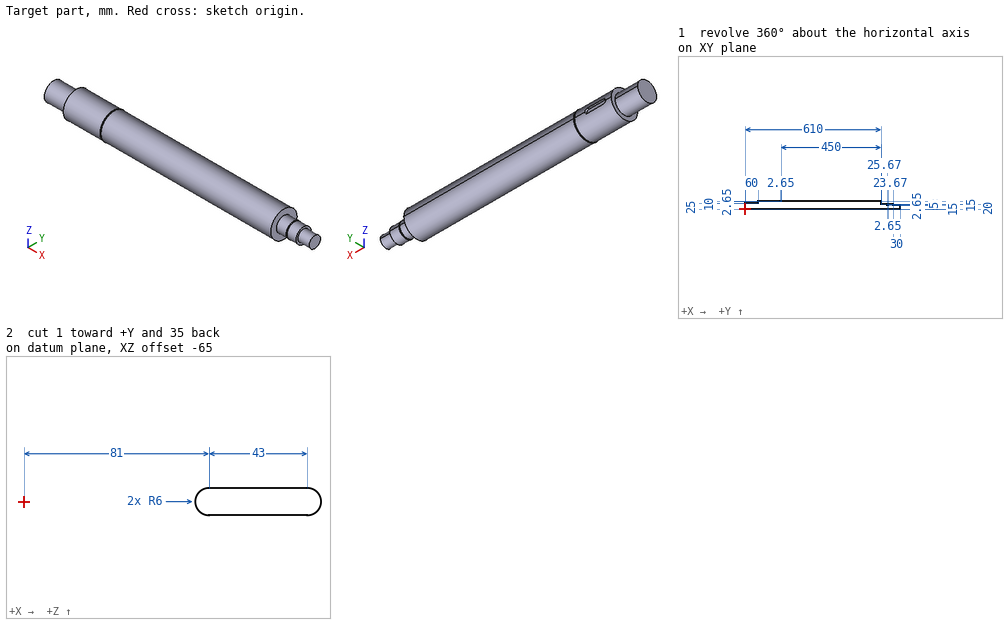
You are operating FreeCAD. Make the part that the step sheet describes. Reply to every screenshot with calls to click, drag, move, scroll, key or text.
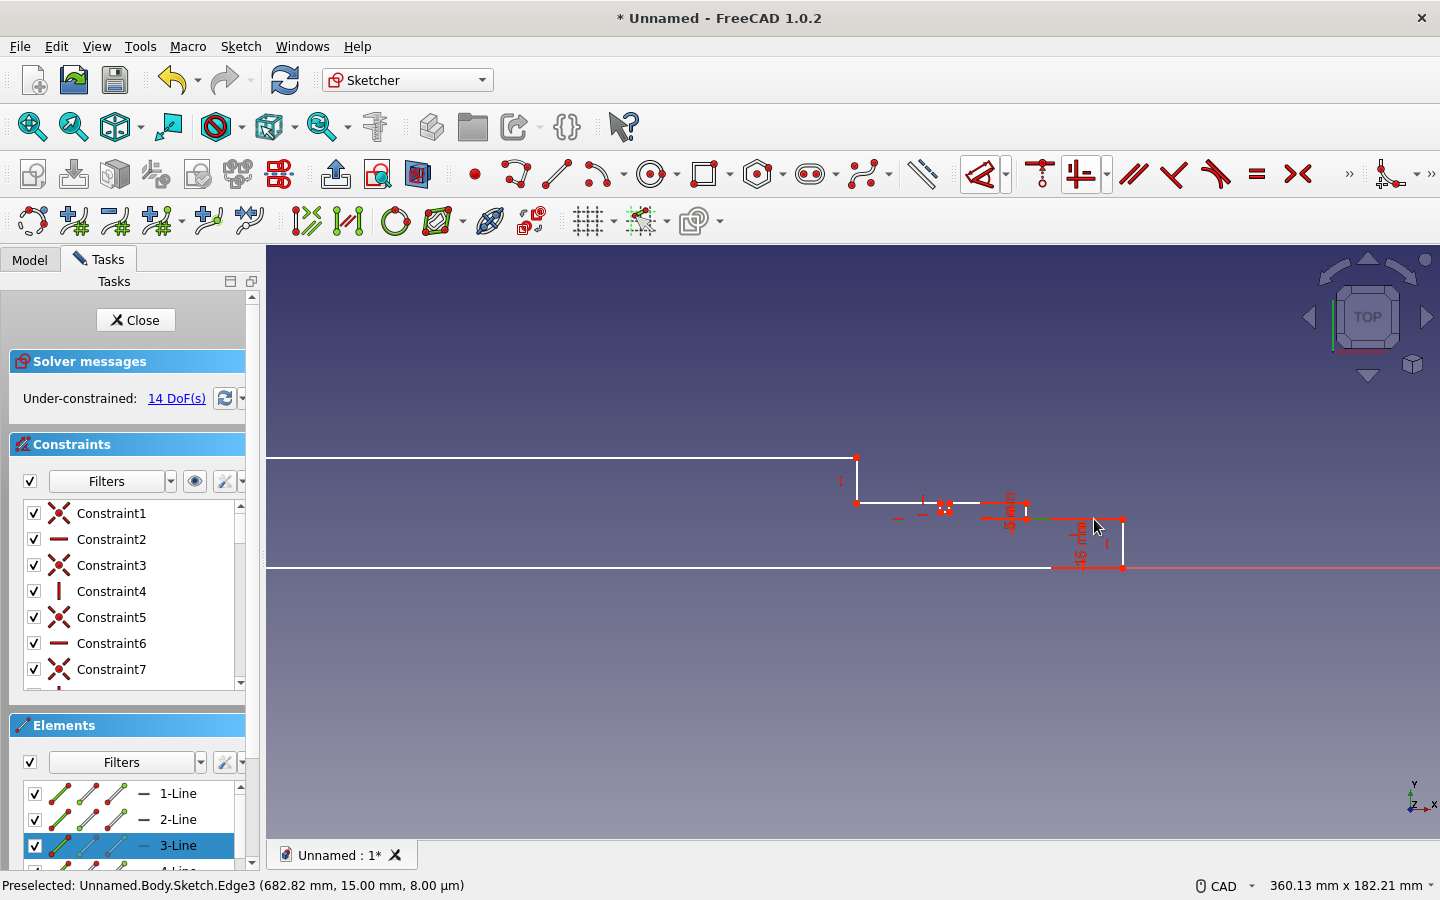
key(l)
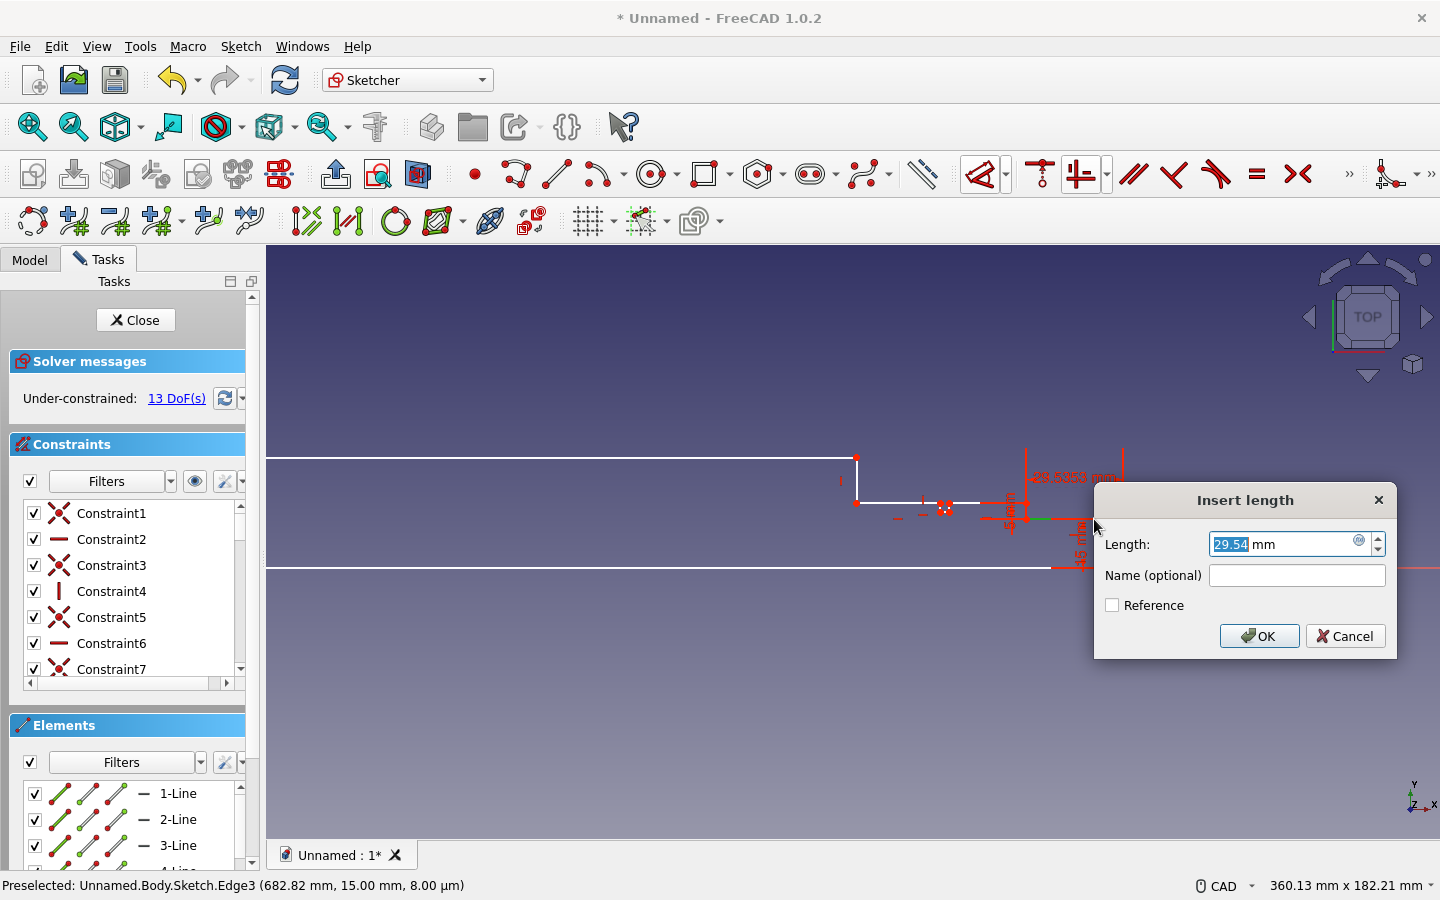
text(30)
key(Return)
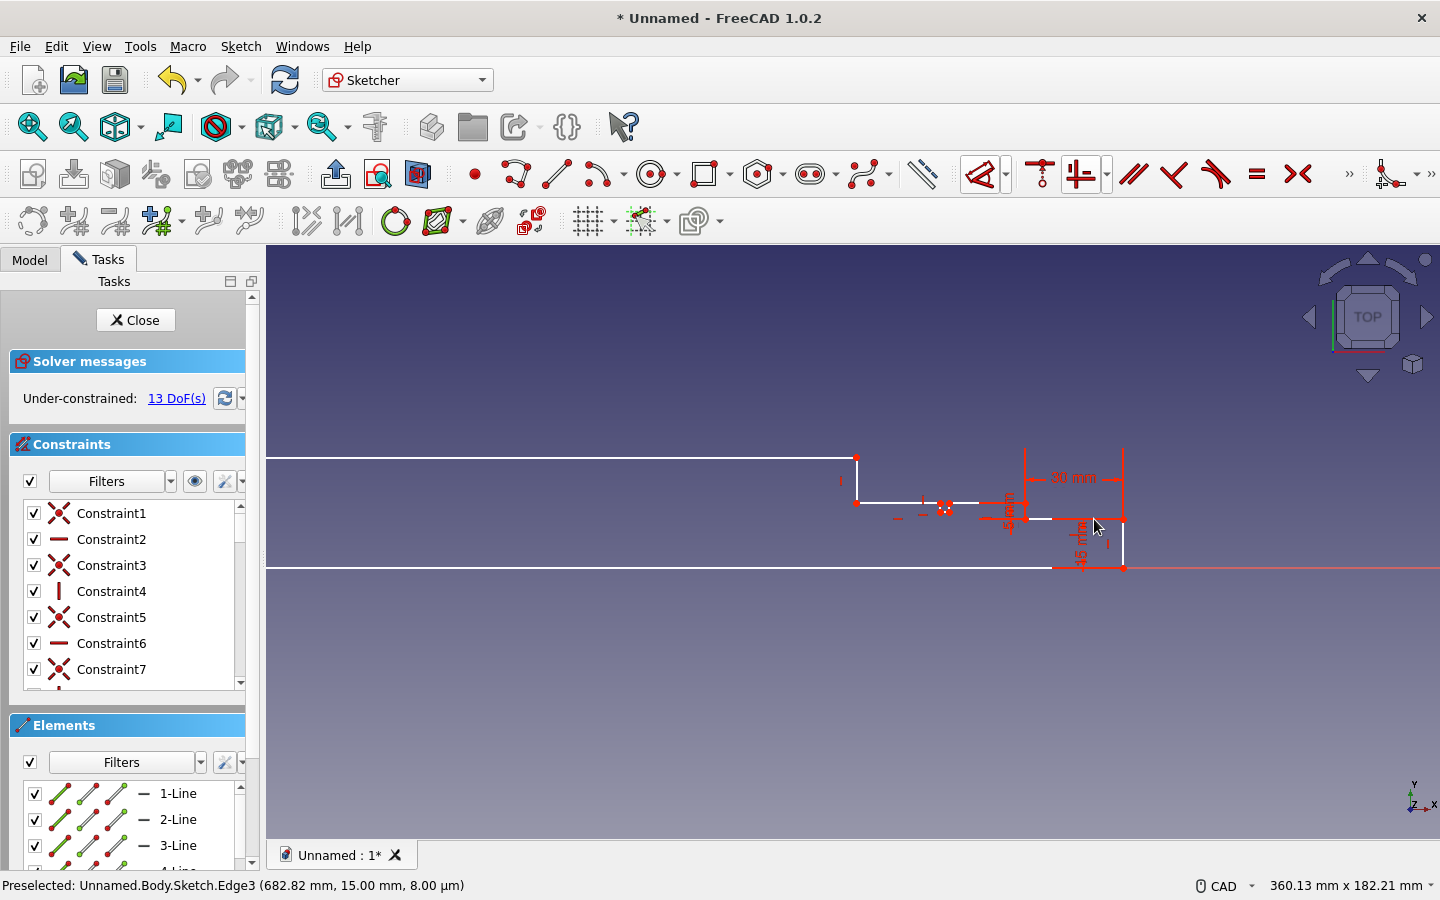
click(857, 490)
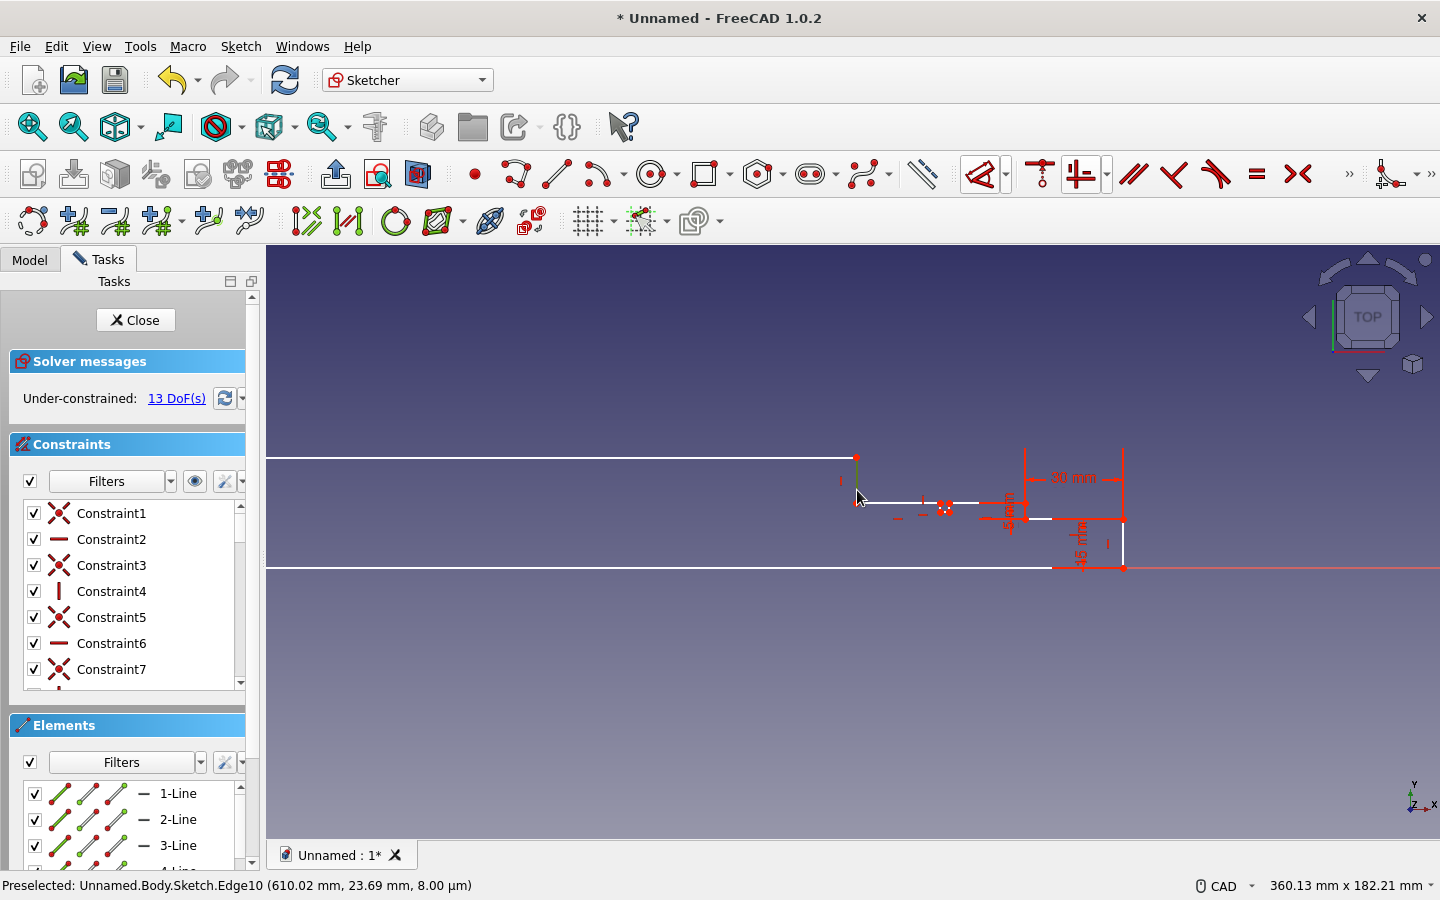
key(i)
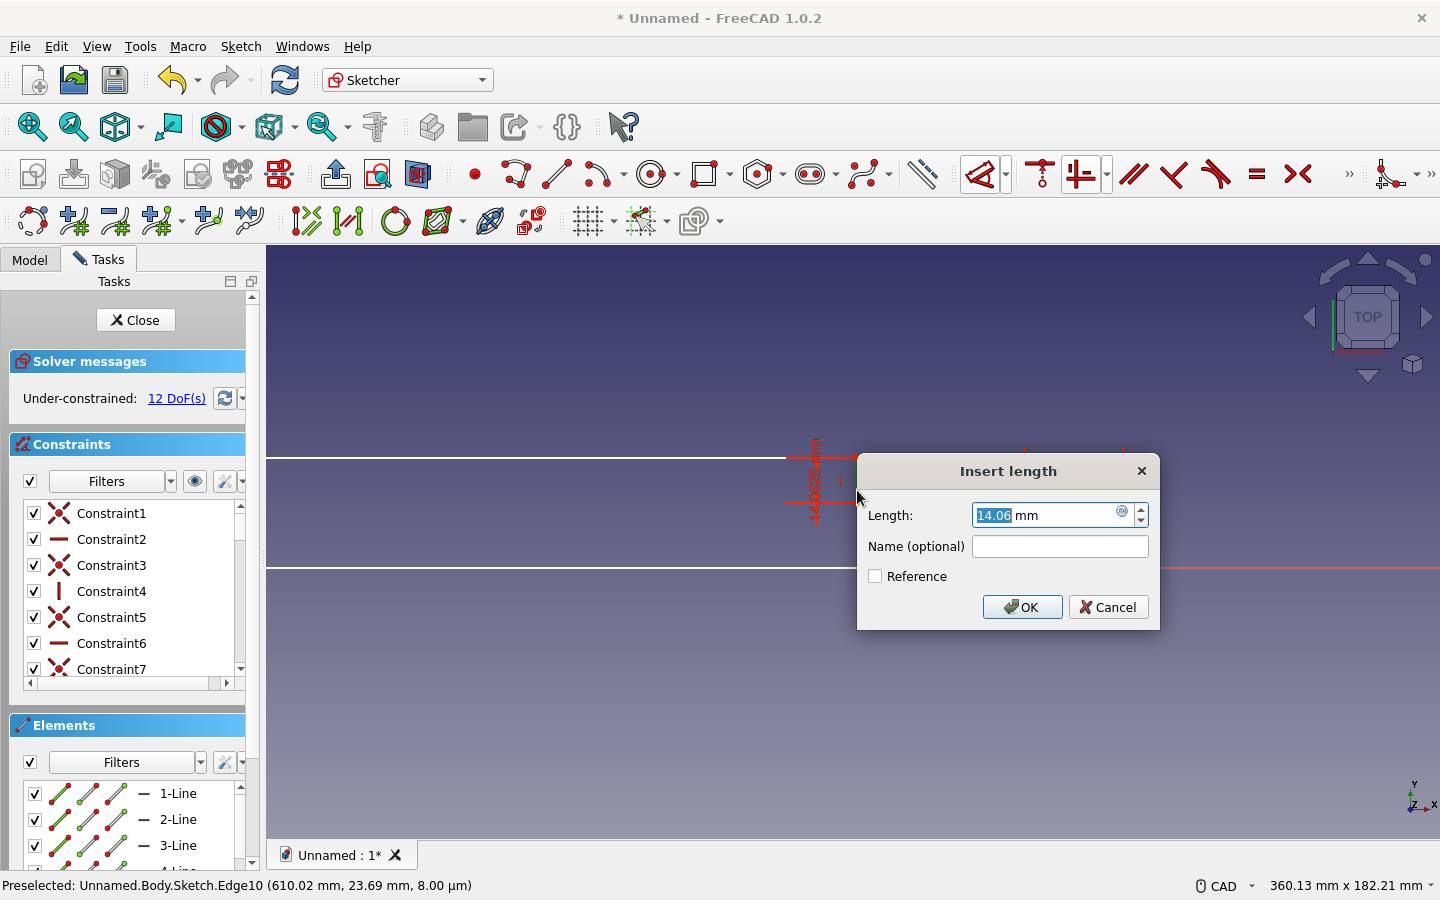
text(15)
key(Return)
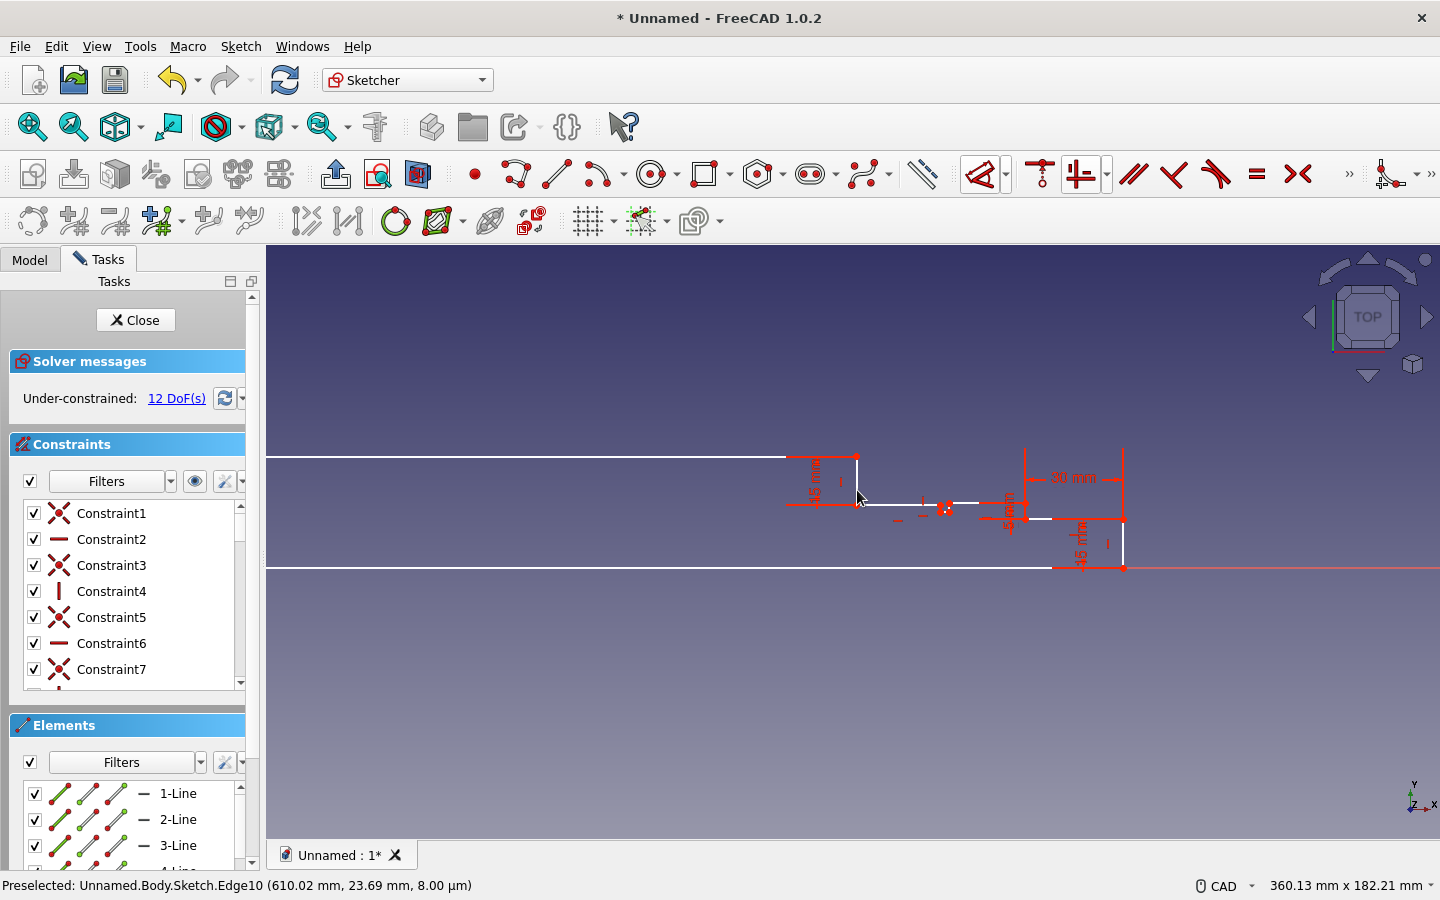
scroll(1124, 555, down, 6)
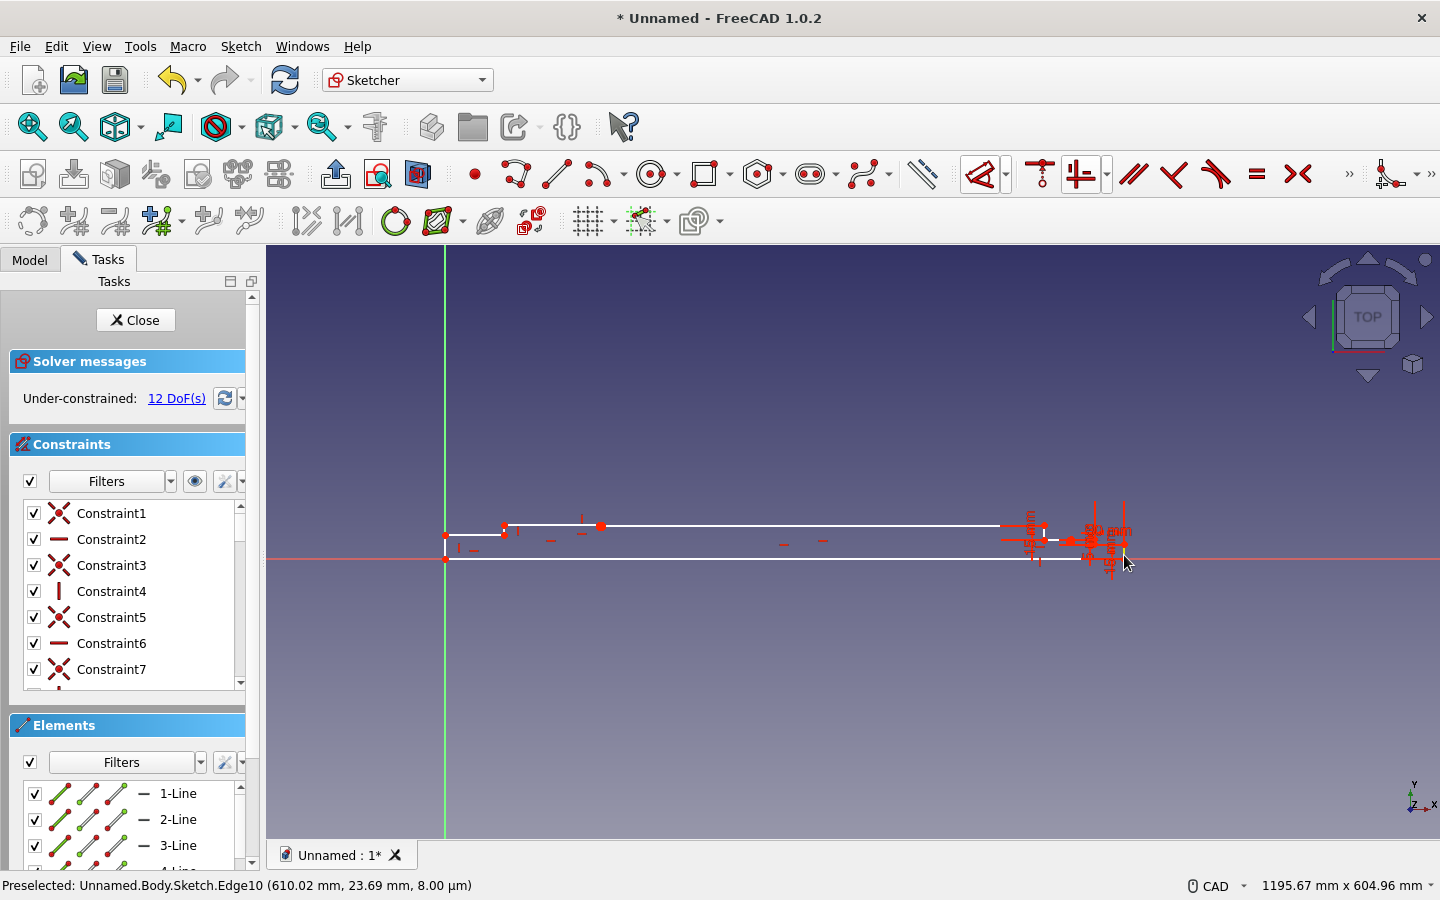
scroll(504, 528, up, 8)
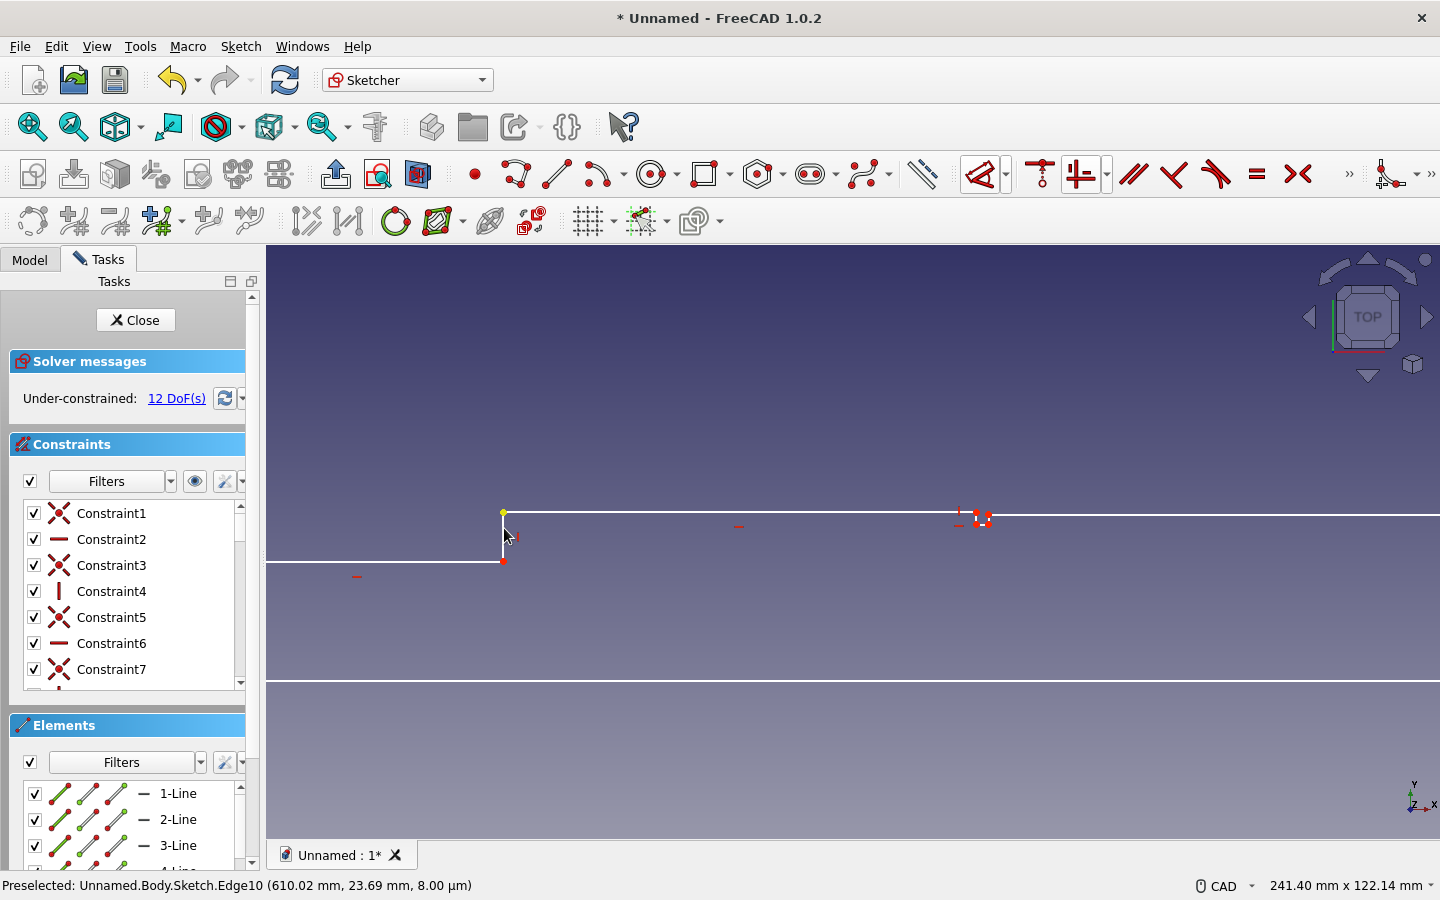
click(503, 527)